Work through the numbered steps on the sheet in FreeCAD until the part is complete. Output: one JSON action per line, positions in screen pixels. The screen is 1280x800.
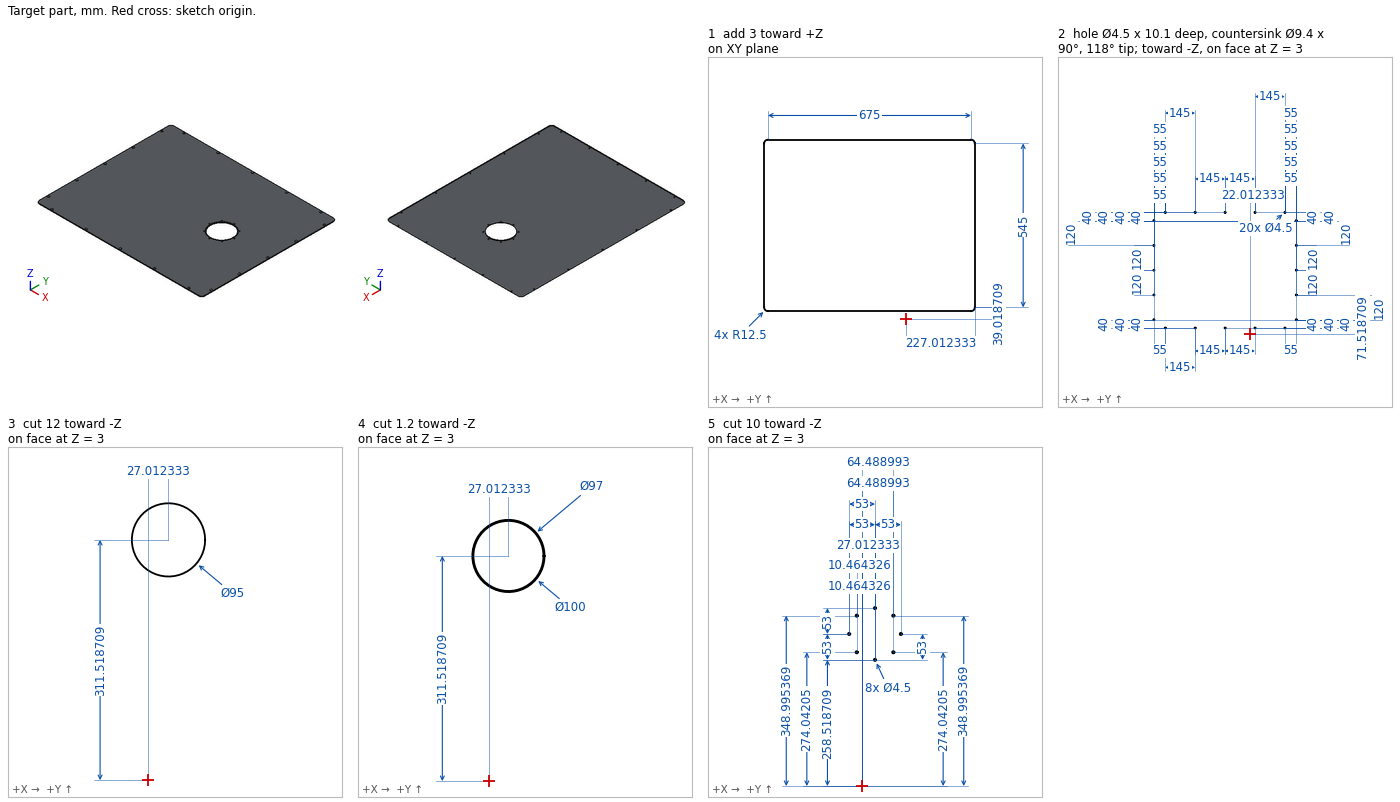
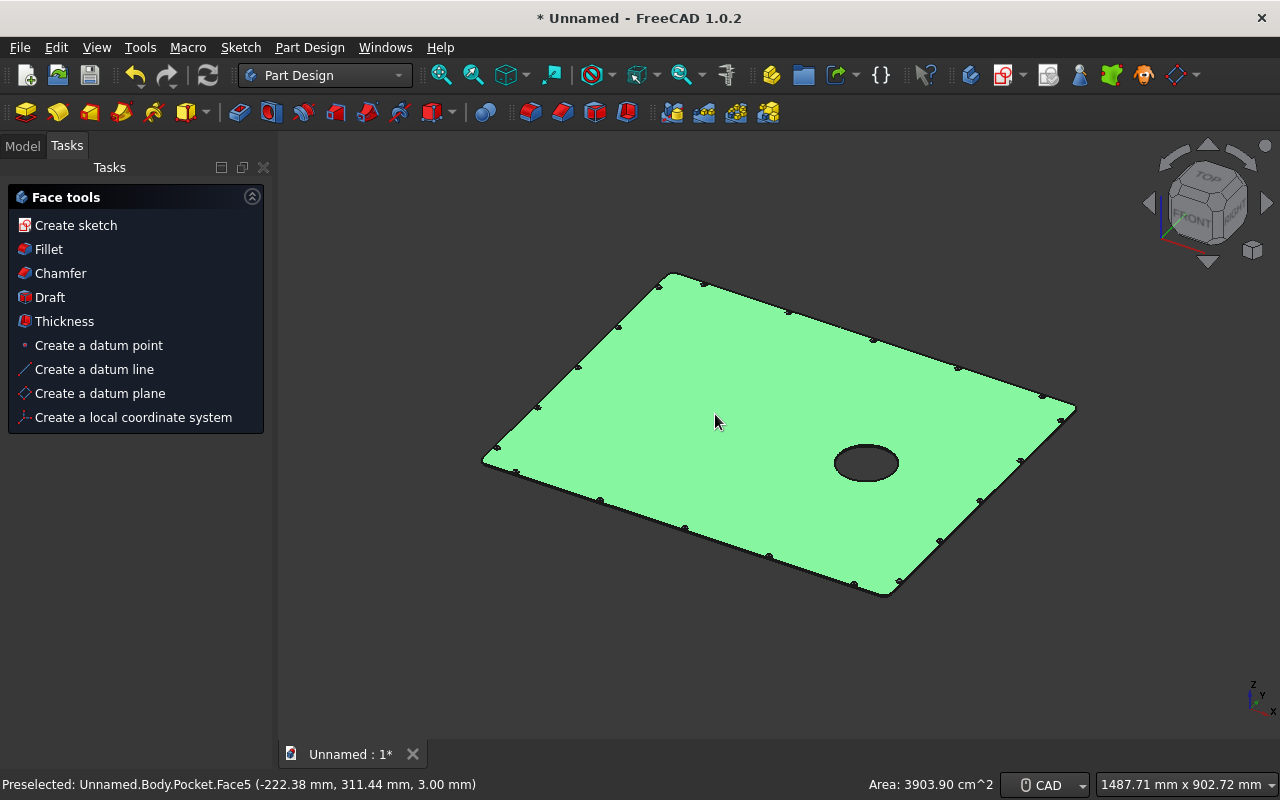
{"action": "left_click", "coordinate": [1004, 76]}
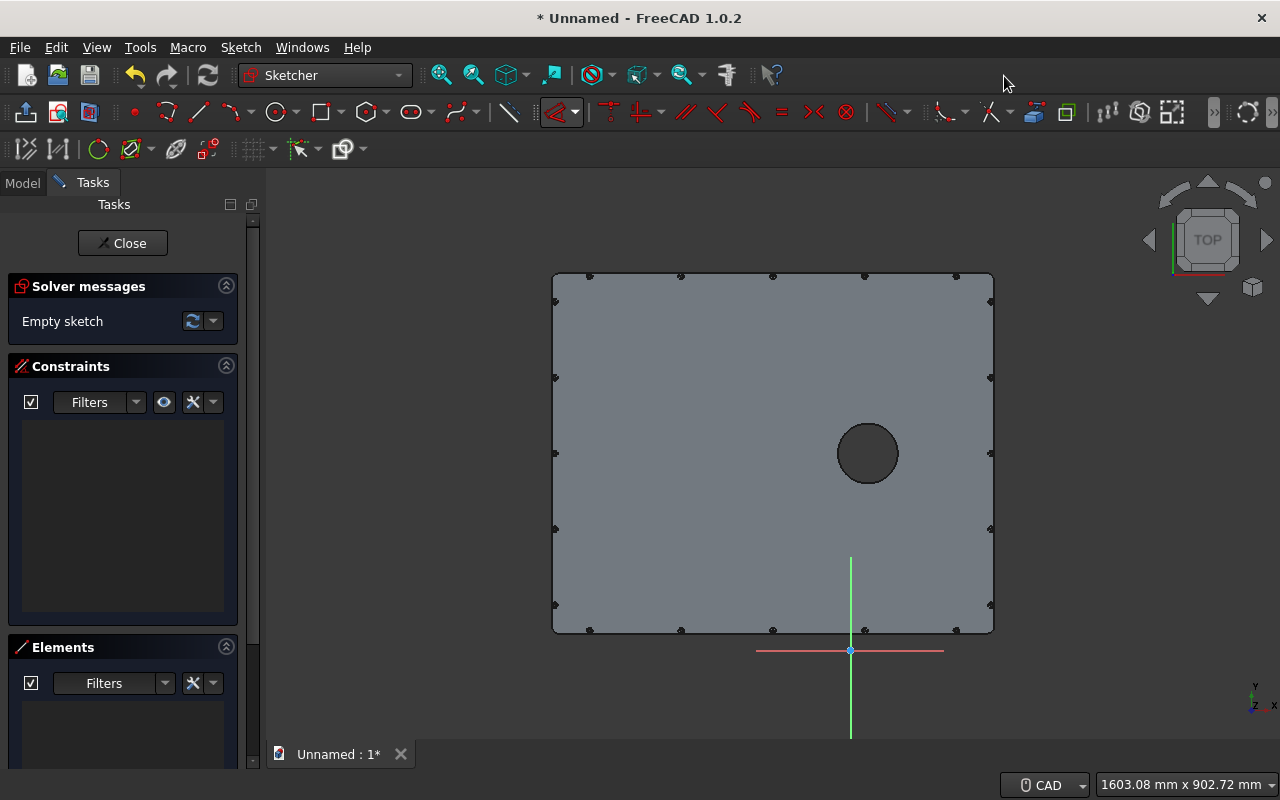
{"action": "scroll", "coordinate": [900, 454], "scroll_direction": "up", "scroll_amount": 9}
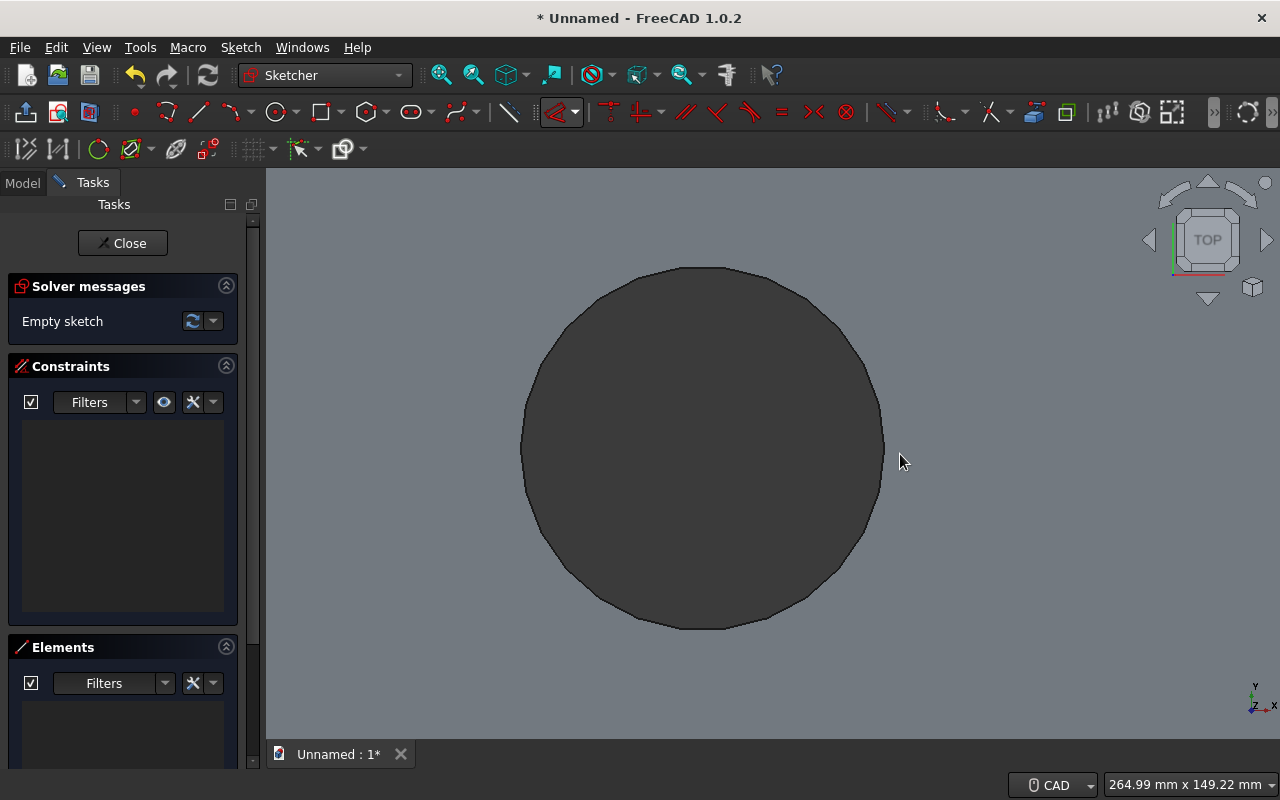
{"action": "left_click", "coordinate": [276, 112]}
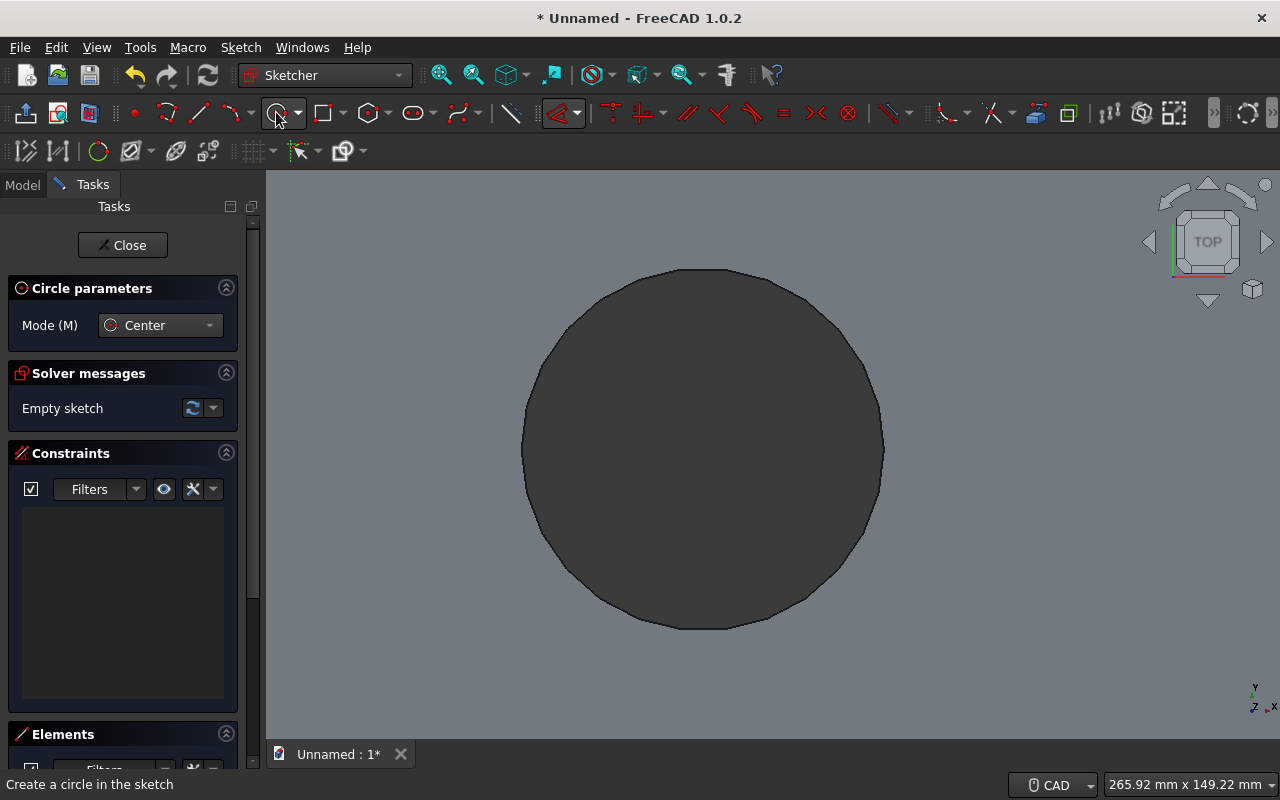
{"action": "left_click", "coordinate": [703, 449]}
{"action": "left_click", "coordinate": [838, 315]}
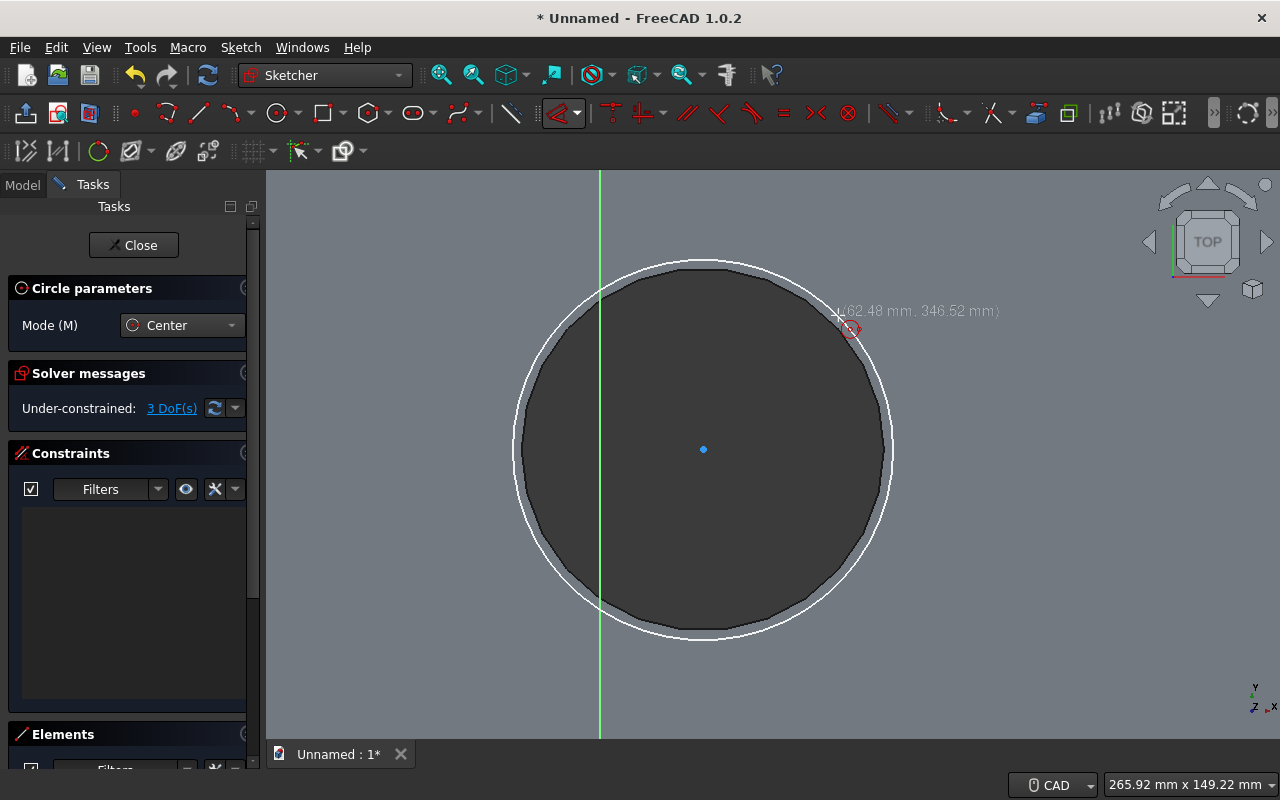
{"action": "left_click", "coordinate": [703, 450]}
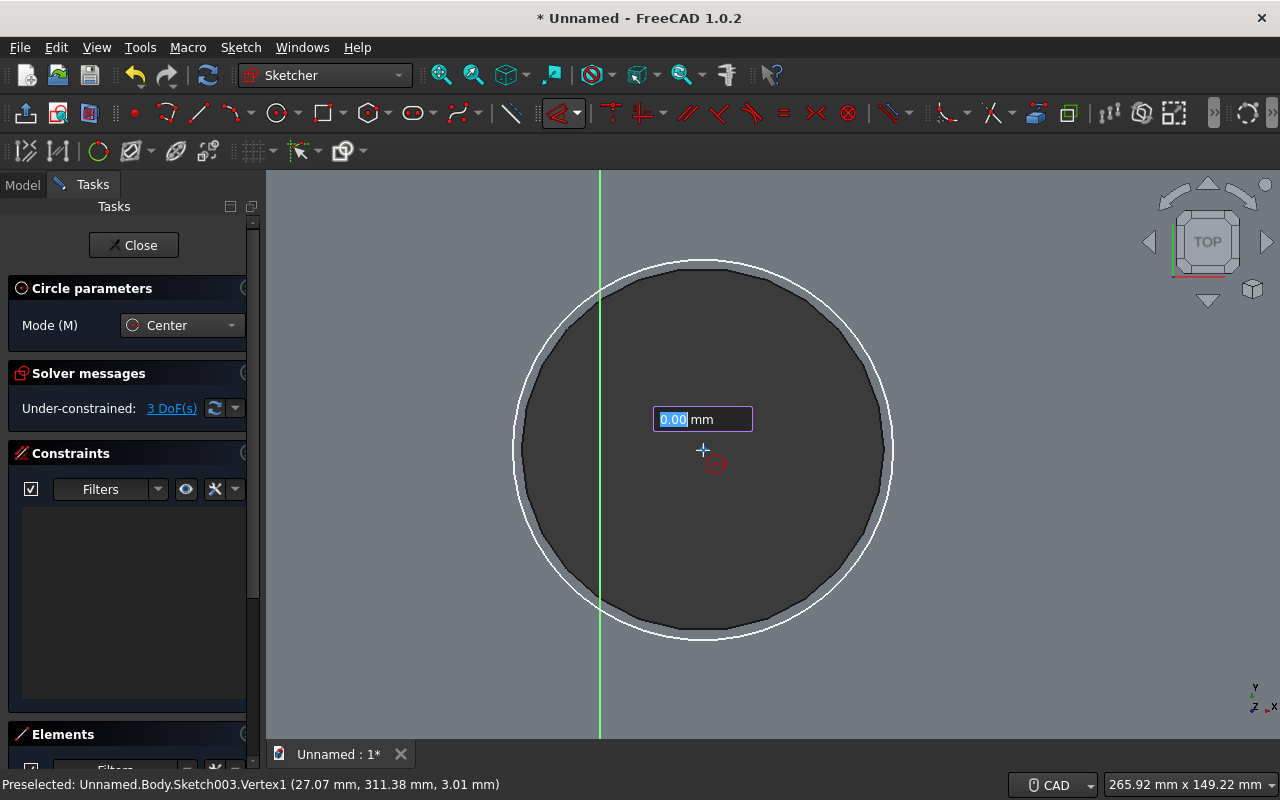
{"action": "scroll", "coordinate": [834, 319], "scroll_direction": "up", "scroll_amount": 6}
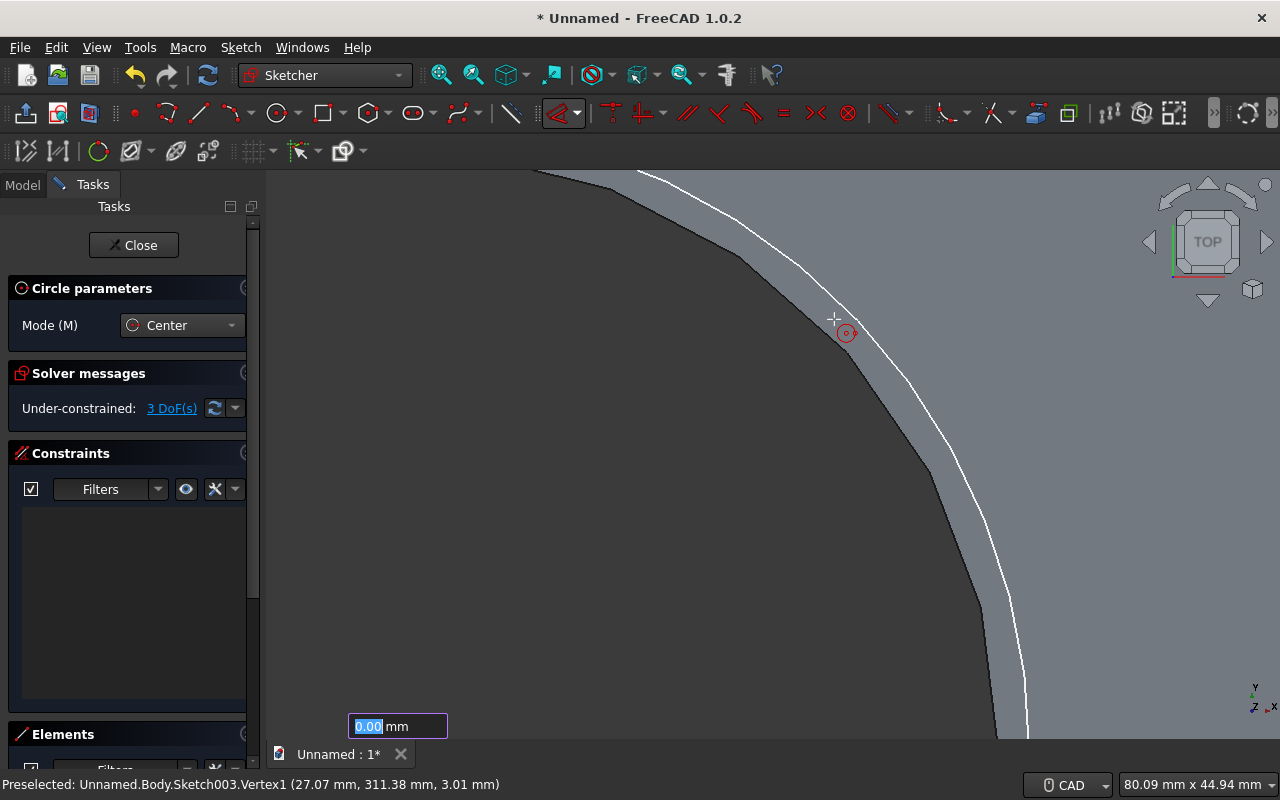
{"action": "left_click", "coordinate": [831, 317]}
{"action": "key", "text": "Escape"}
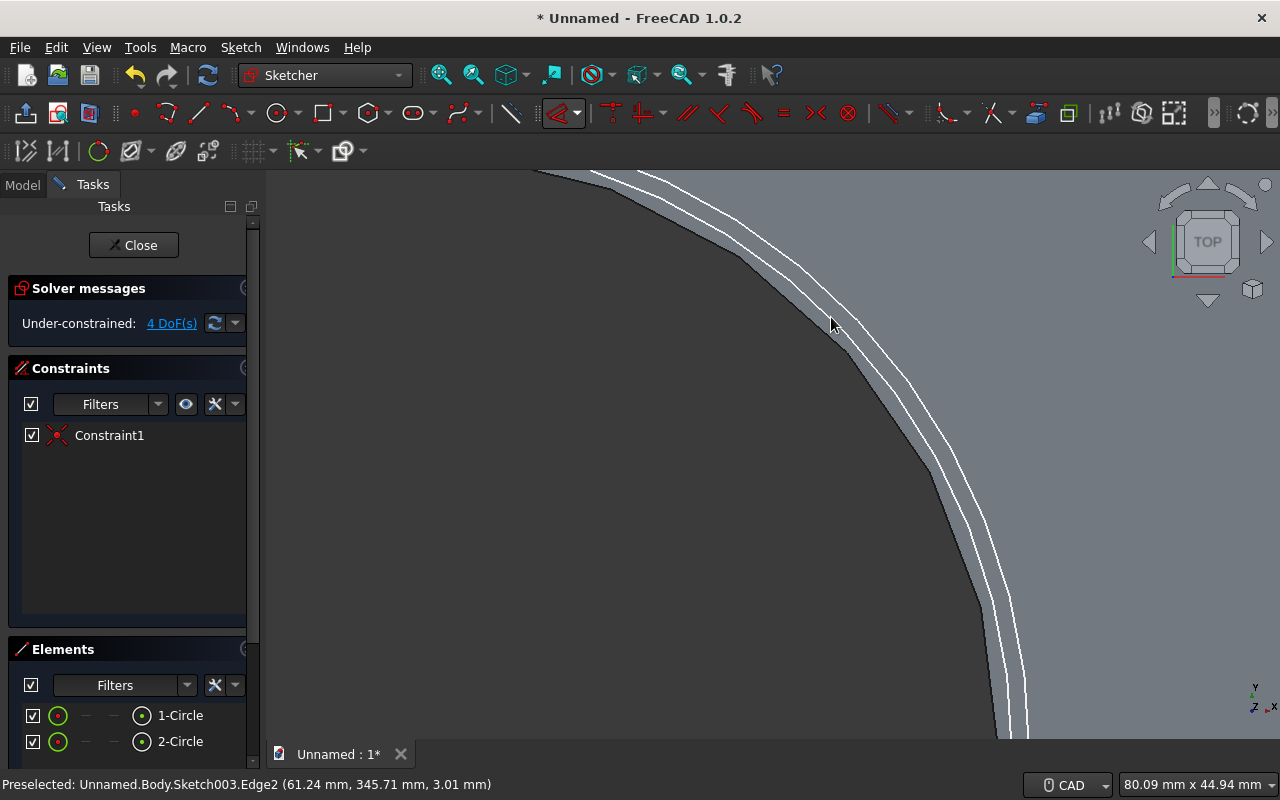
{"action": "left_click", "coordinate": [843, 305]}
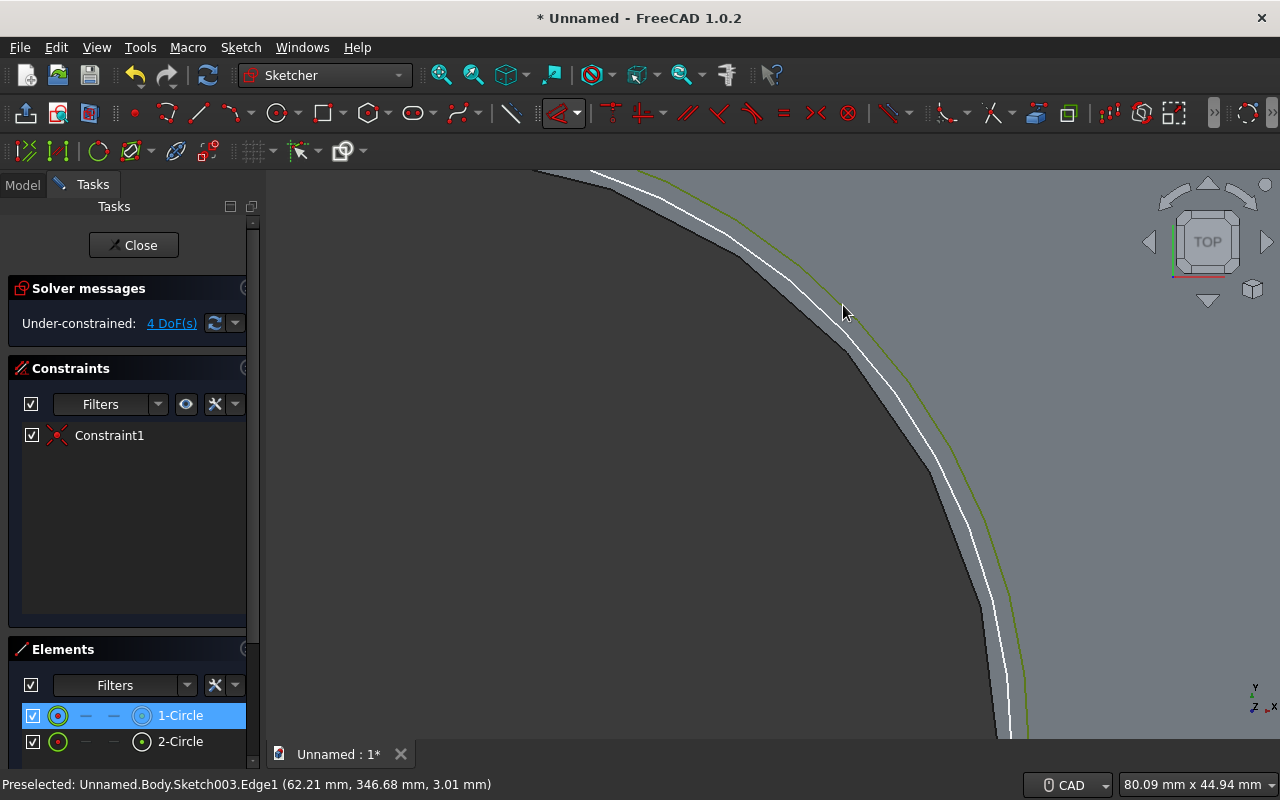
{"action": "key", "text": "k o"}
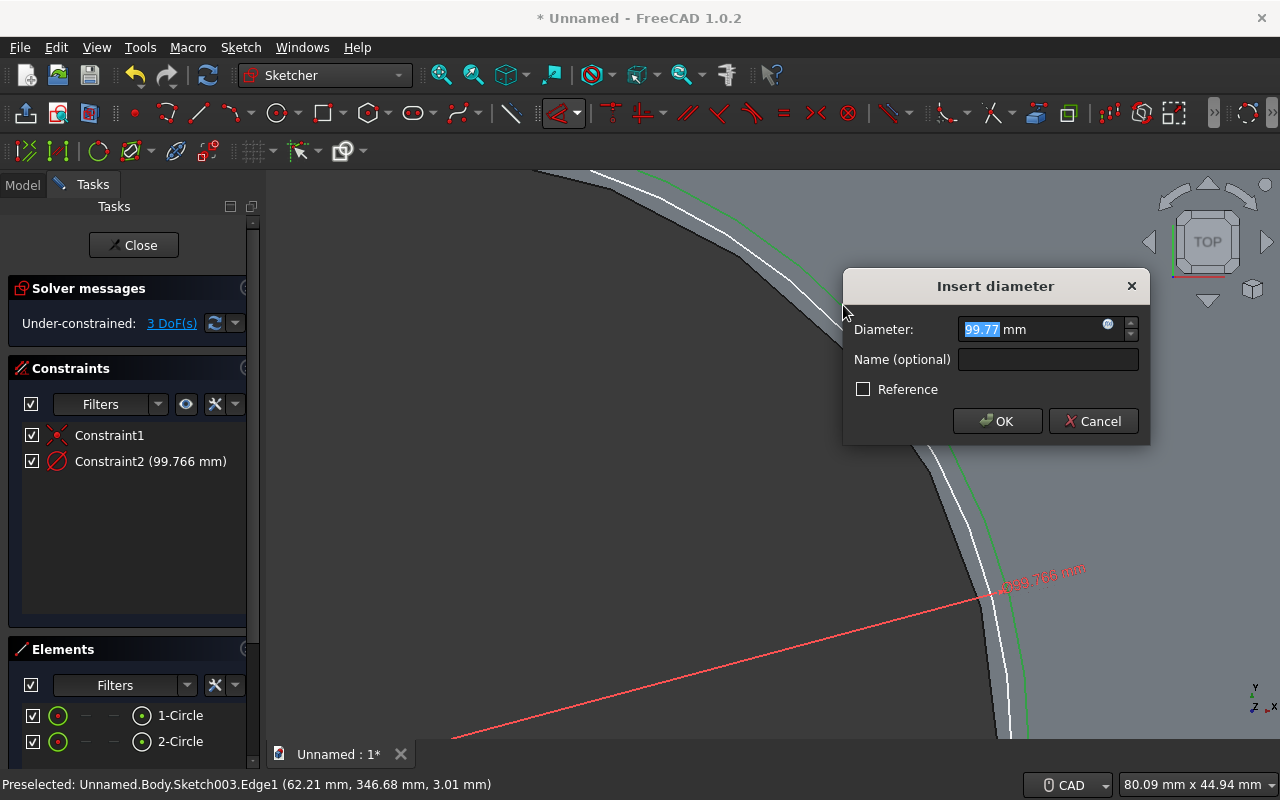
{"action": "type", "text": "100"}
{"action": "key", "text": "Return"}